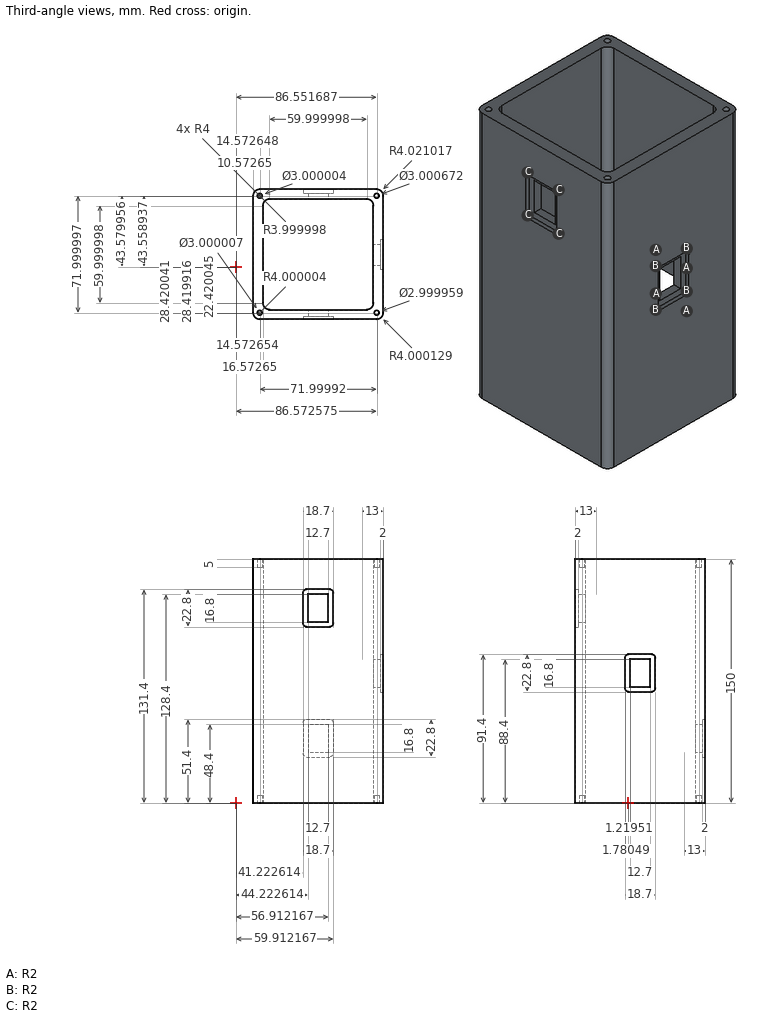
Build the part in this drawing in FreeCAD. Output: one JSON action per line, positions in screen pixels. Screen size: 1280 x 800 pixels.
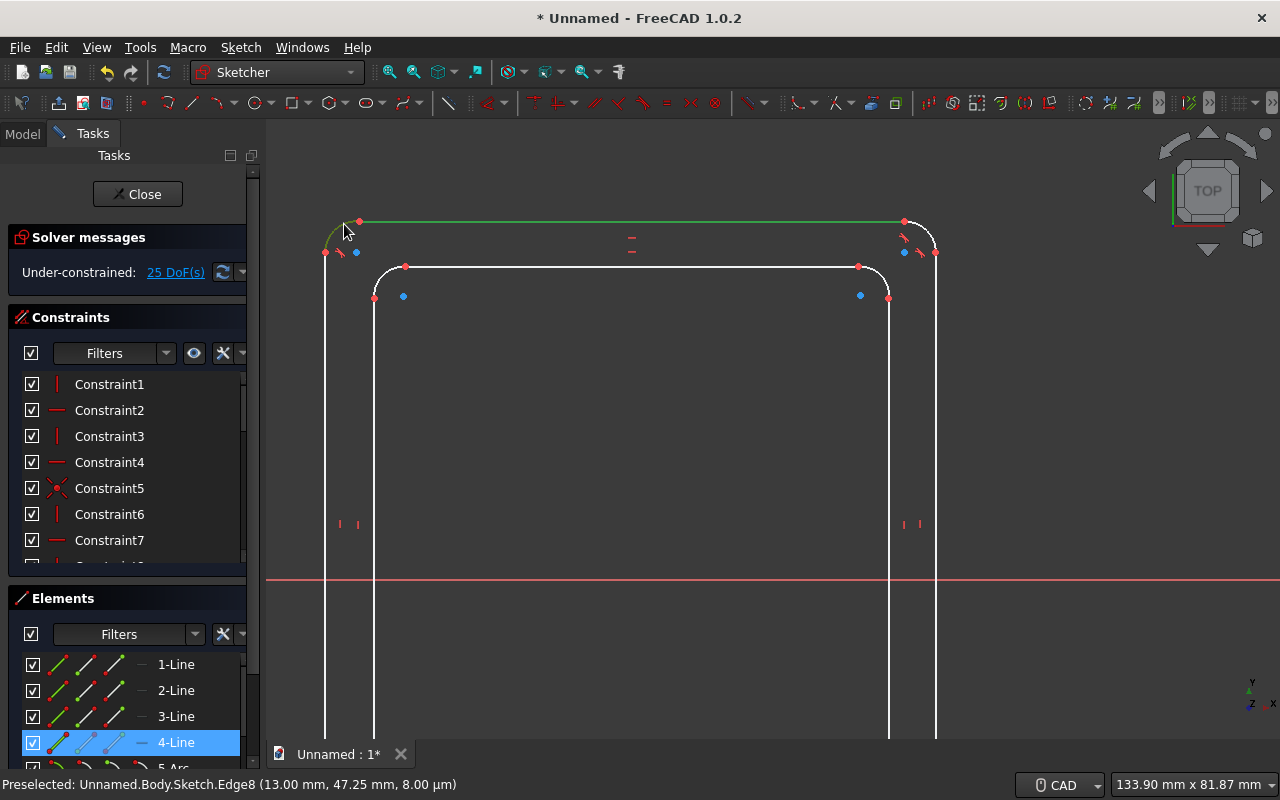
{"action": "left_click", "coordinate": [644, 104]}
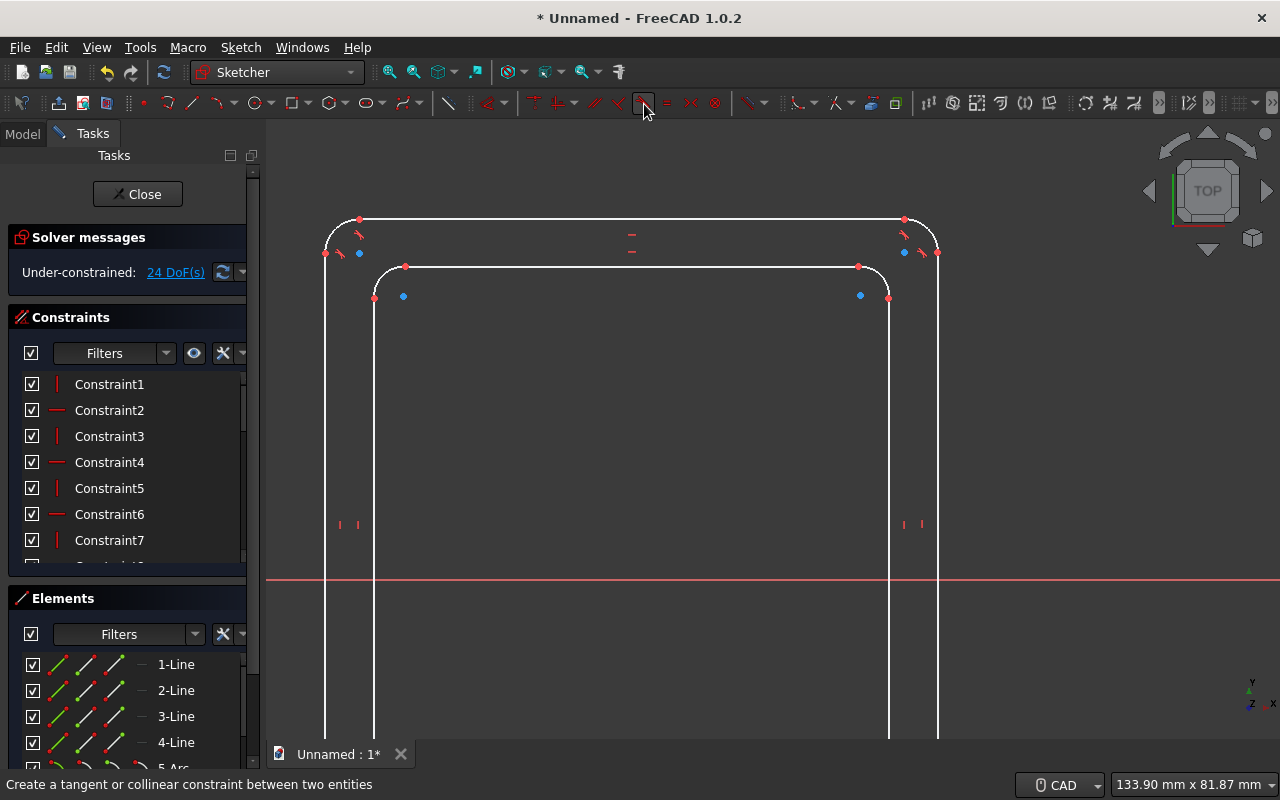
{"action": "left_click", "coordinate": [374, 615]}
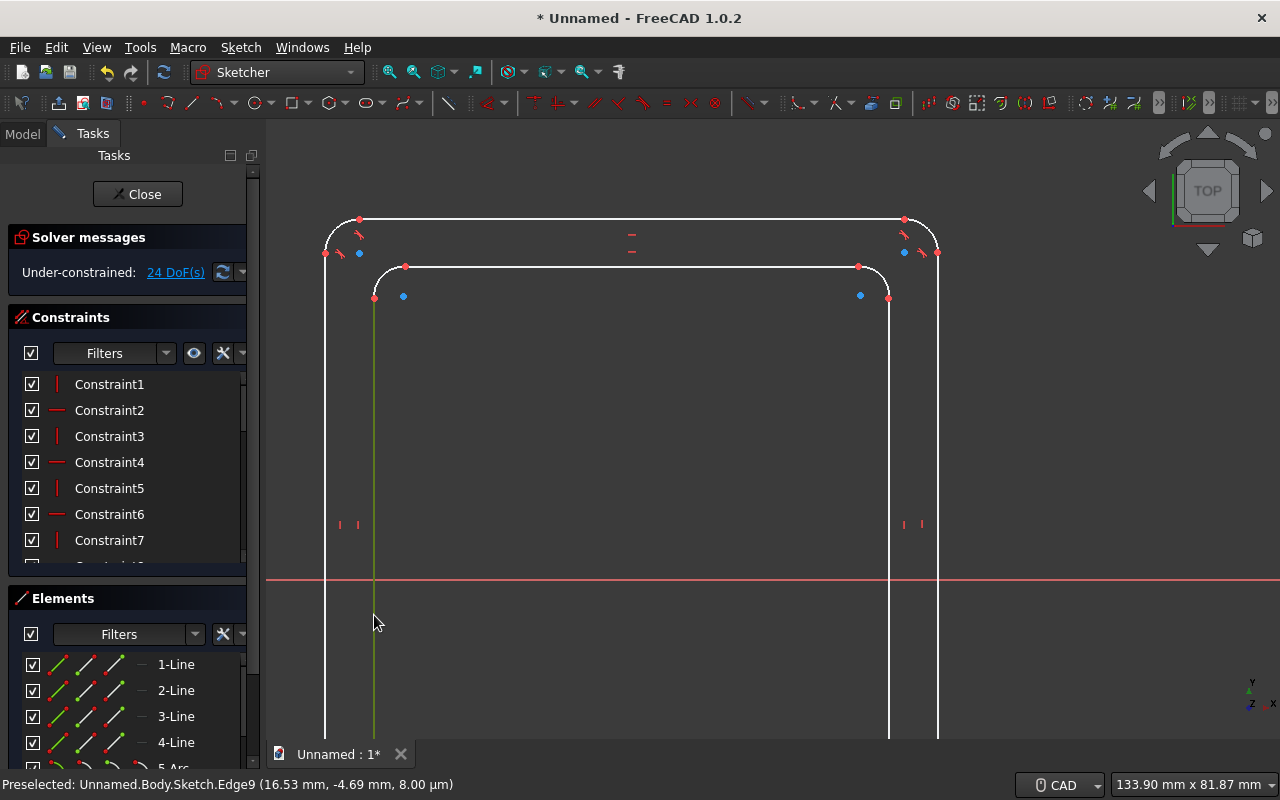
{"action": "left_click", "coordinate": [391, 270]}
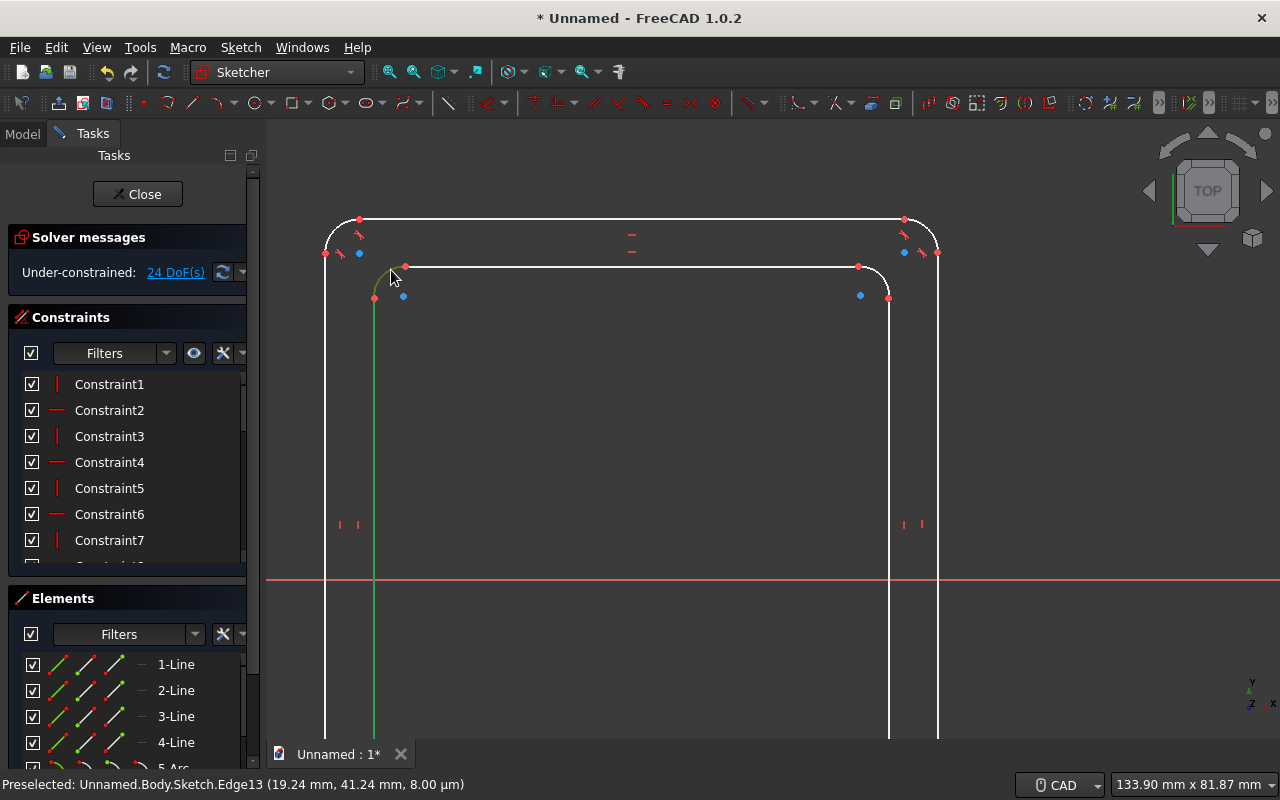
{"action": "key", "text": "t"}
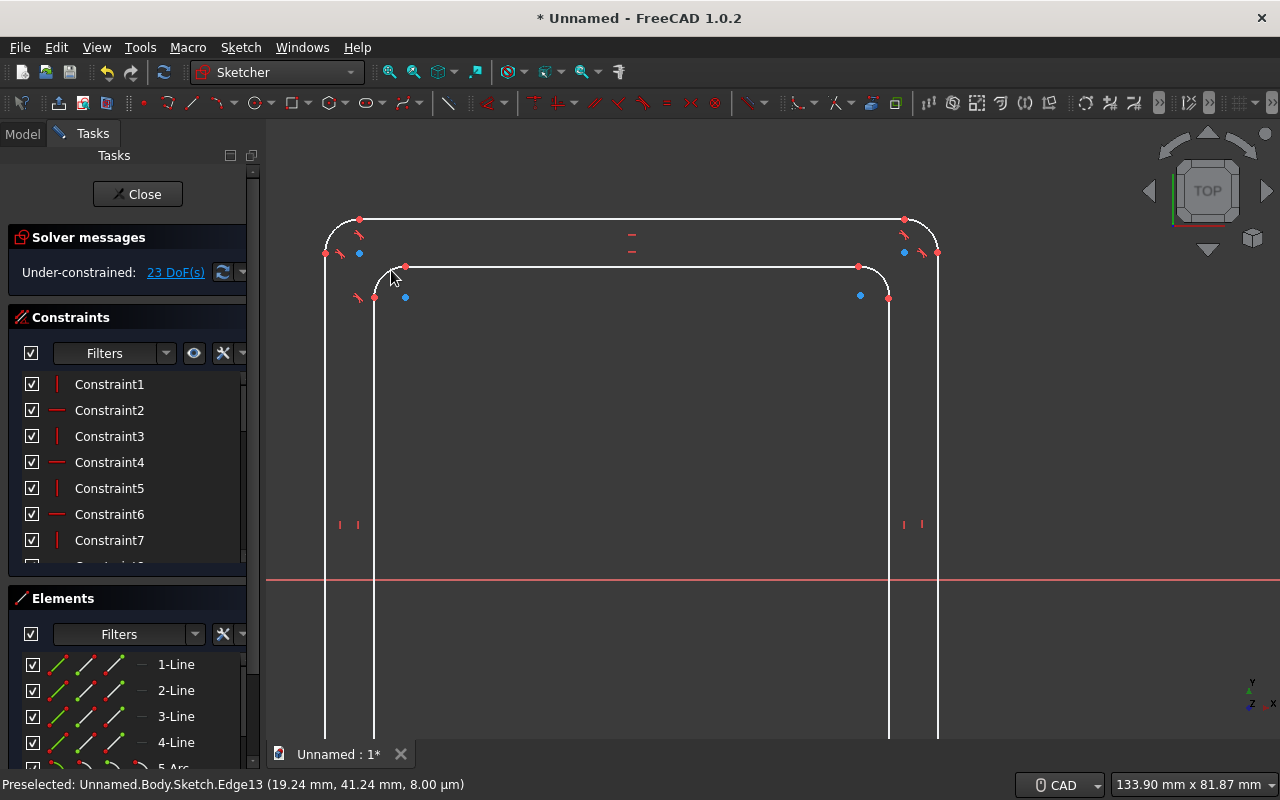
{"action": "left_click", "coordinate": [374, 615]}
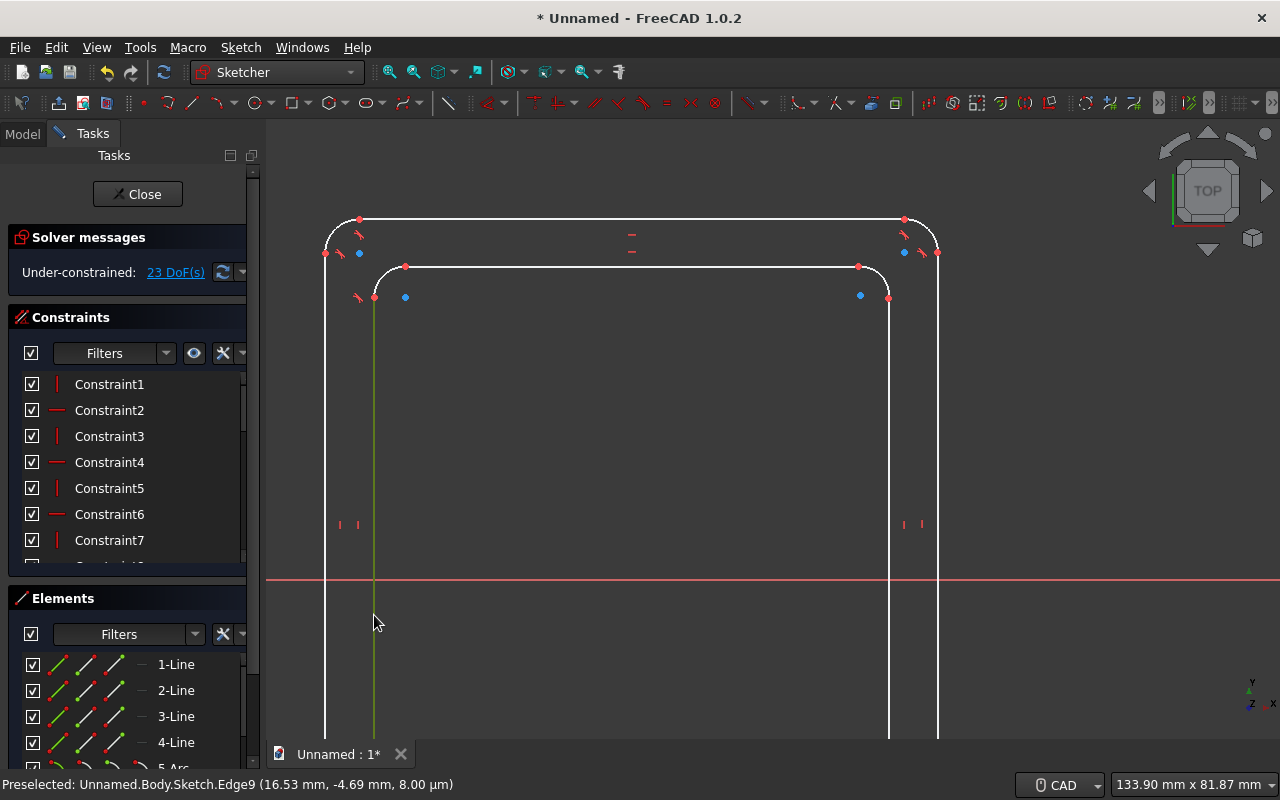
{"action": "scroll", "coordinate": [933, 238], "scroll_direction": "down", "scroll_amount": 2}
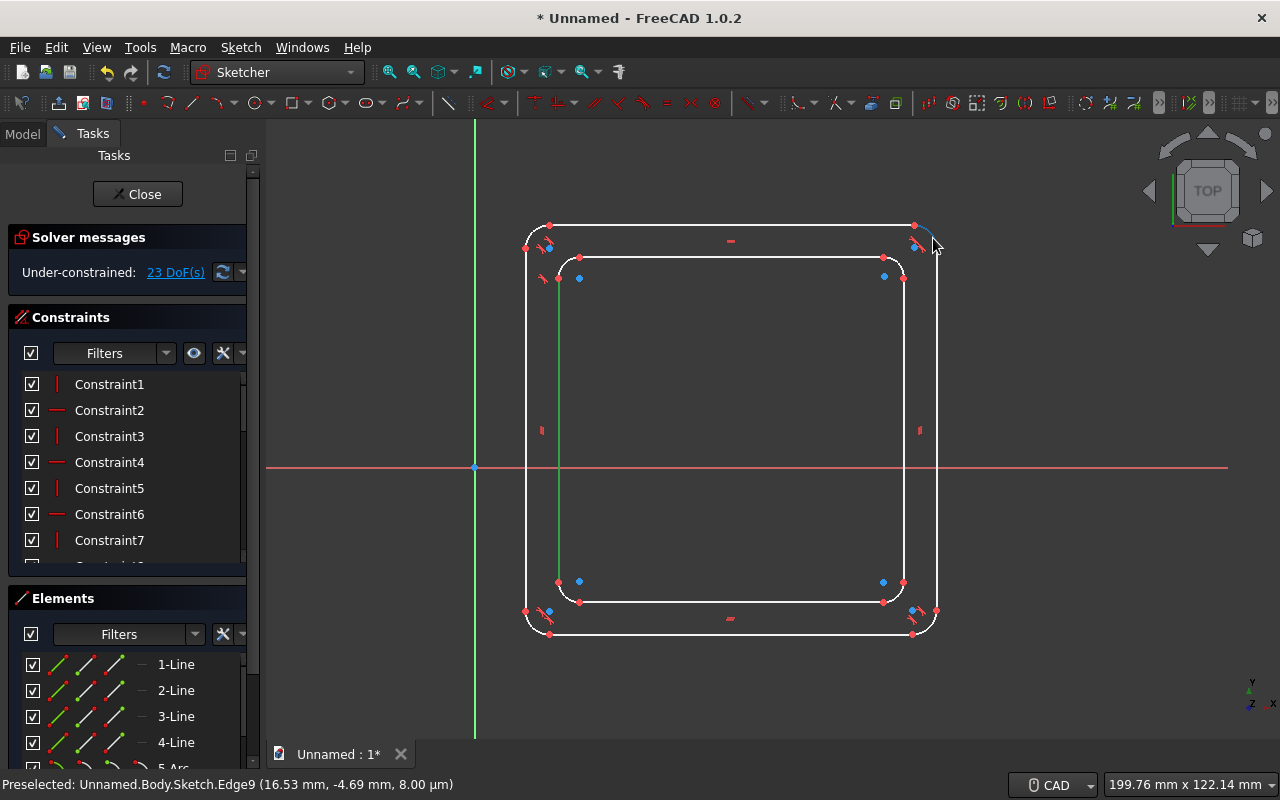
{"action": "scroll", "coordinate": [561, 591], "scroll_direction": "up", "scroll_amount": 2}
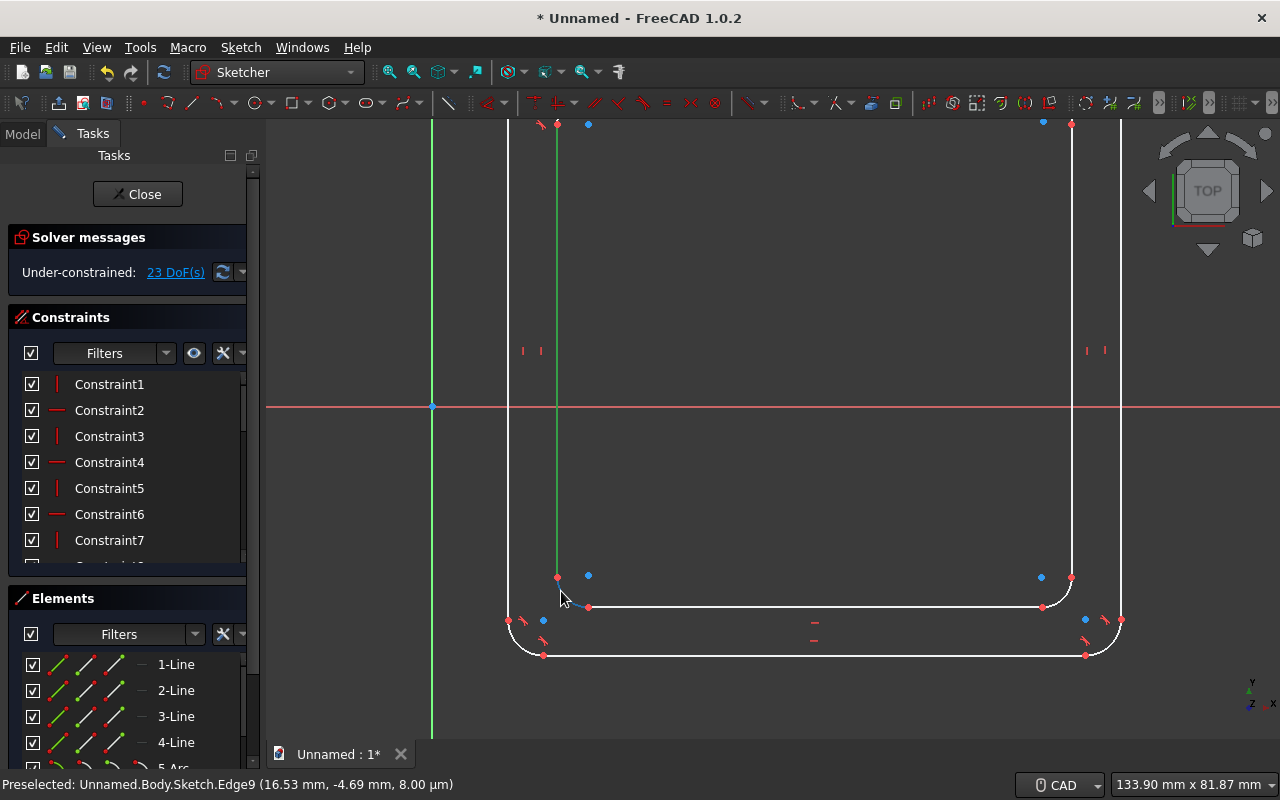
{"action": "left_click", "coordinate": [561, 591]}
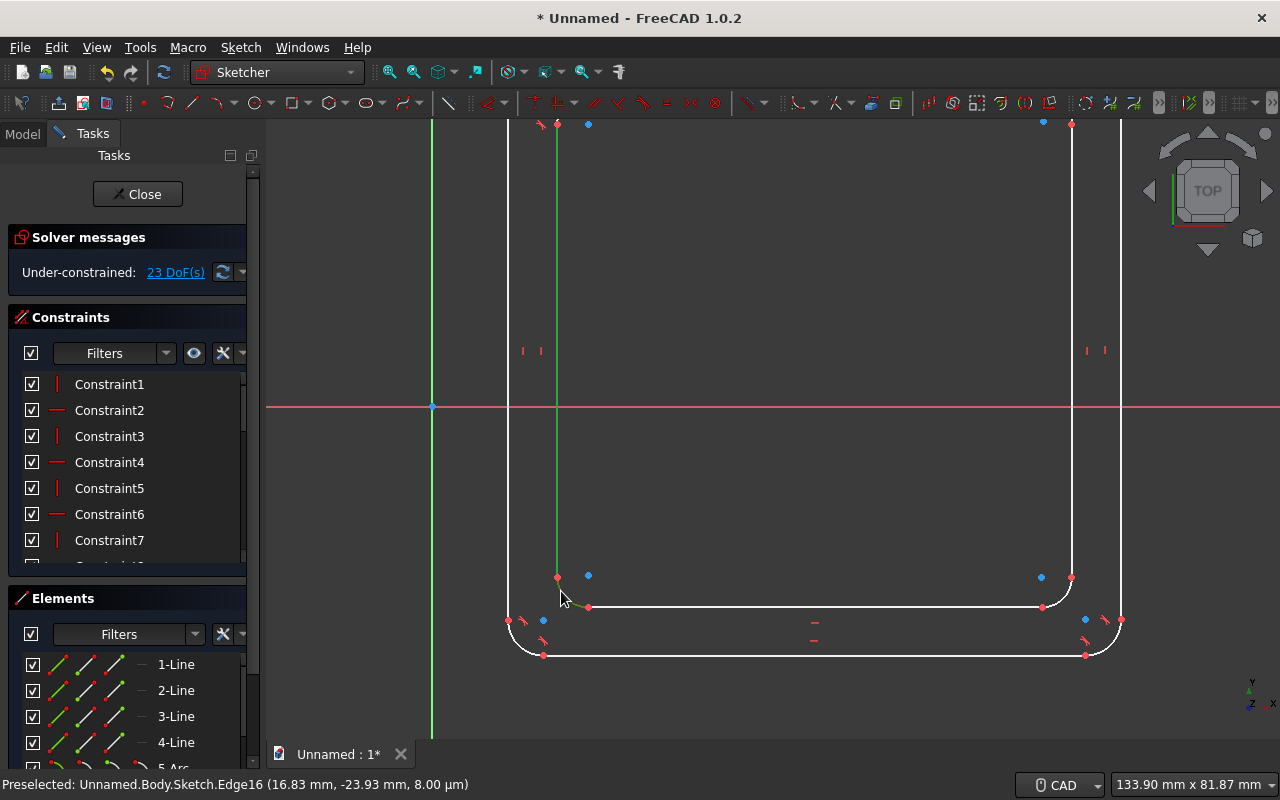
{"action": "left_click", "coordinate": [644, 104]}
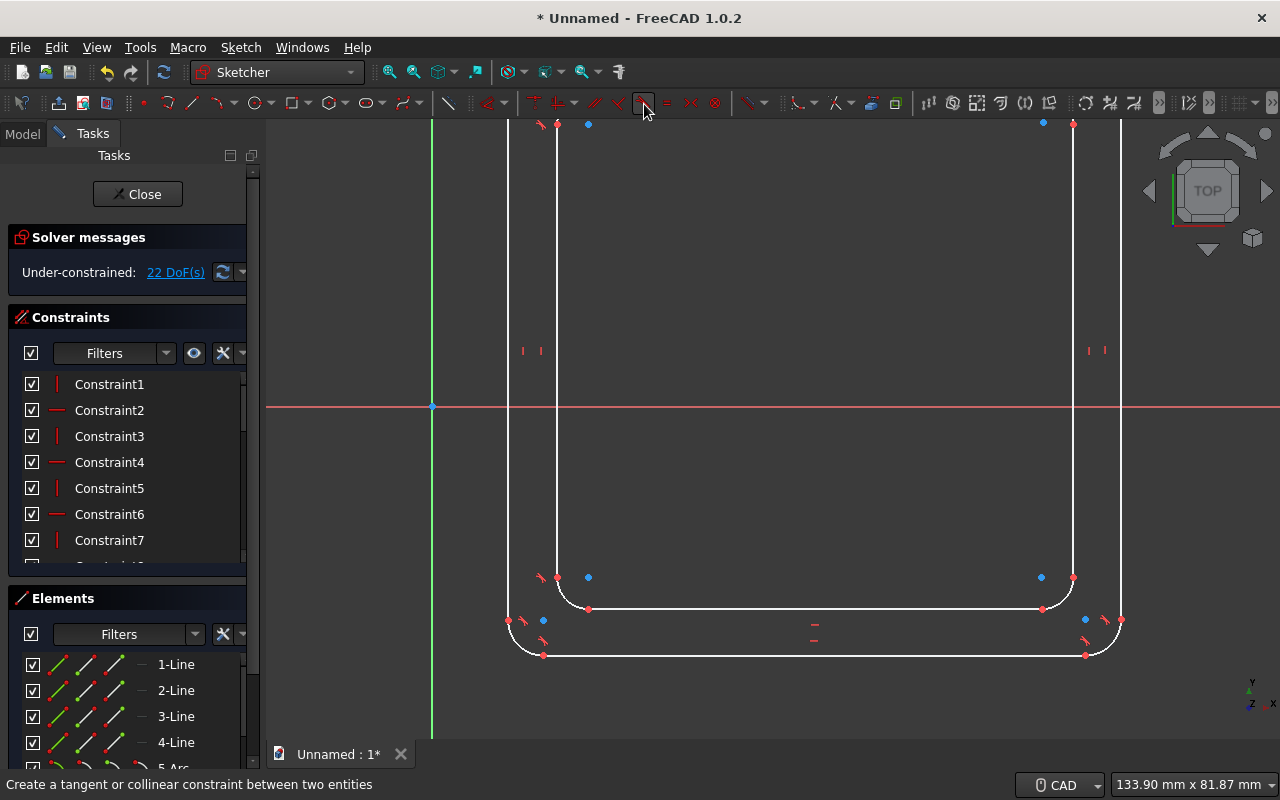
{"action": "scroll", "coordinate": [561, 591], "scroll_direction": "down", "scroll_amount": 2}